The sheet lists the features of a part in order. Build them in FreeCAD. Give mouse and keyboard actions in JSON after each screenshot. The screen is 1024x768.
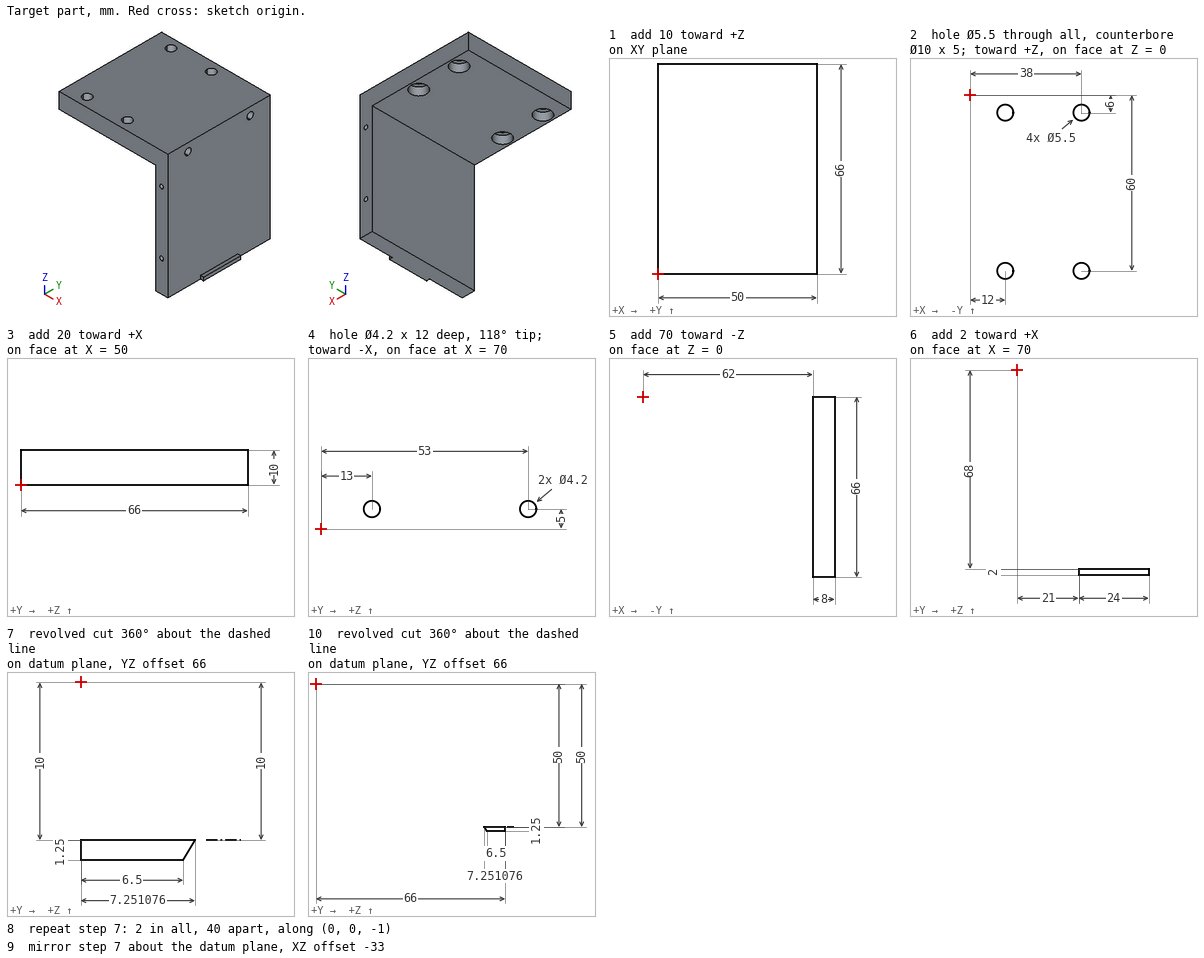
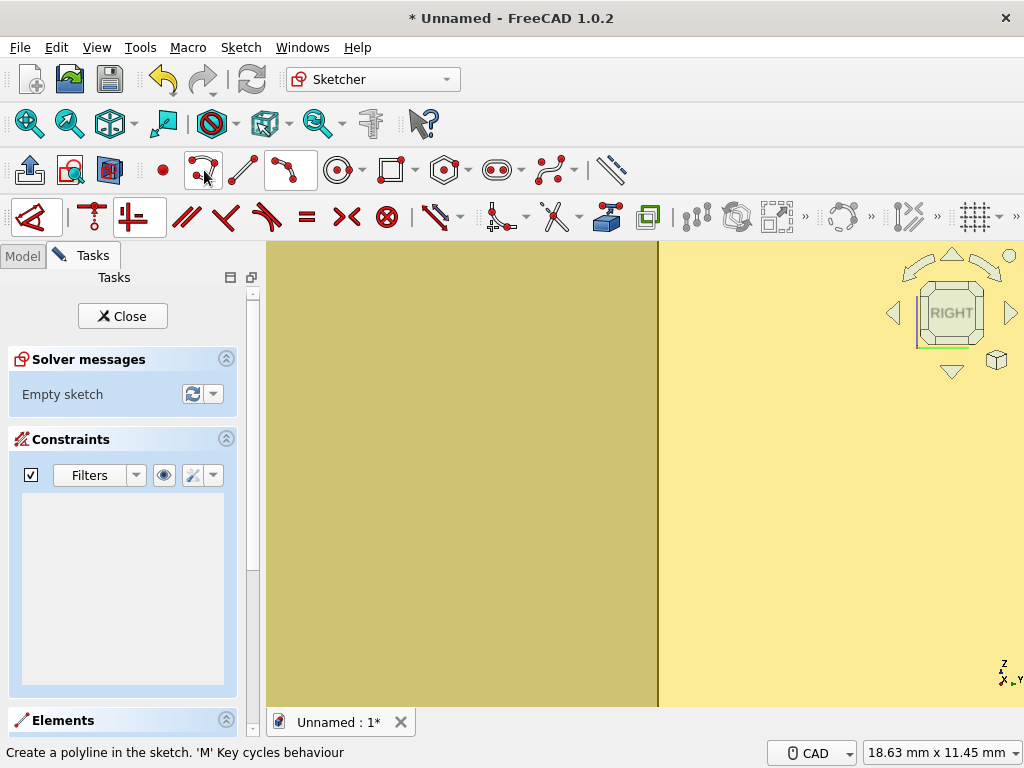
{"action": "left_click", "coordinate": [363, 439]}
{"action": "left_click", "coordinate": [393, 490]}
{"action": "left_click", "coordinate": [658, 490]}
{"action": "left_click", "coordinate": [658, 439]}
{"action": "left_click", "coordinate": [363, 440]}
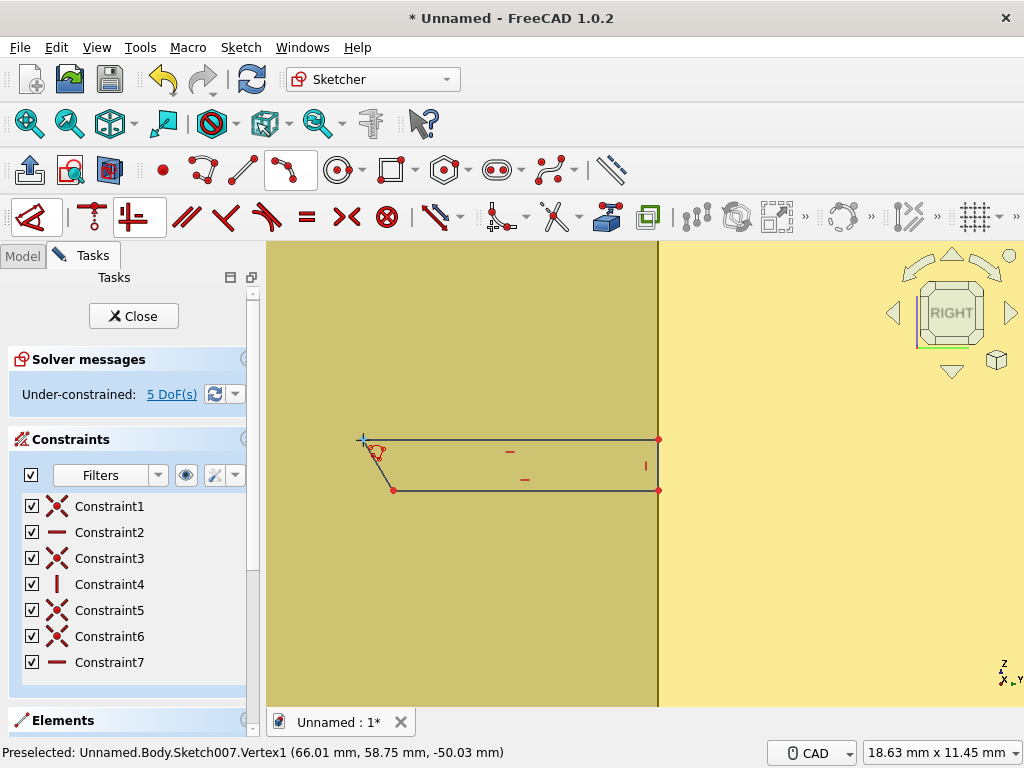
{"action": "key", "text": "g l"}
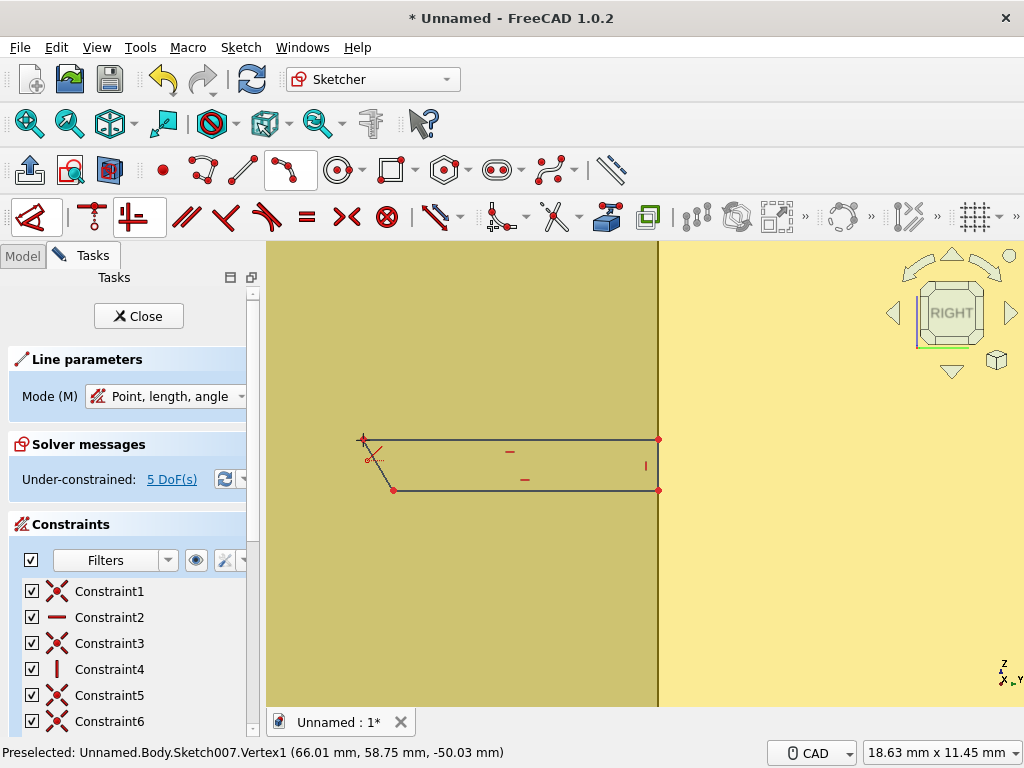
{"action": "left_click", "coordinate": [687, 439]}
{"action": "left_click", "coordinate": [776, 439]}
{"action": "key", "text": "Escape"}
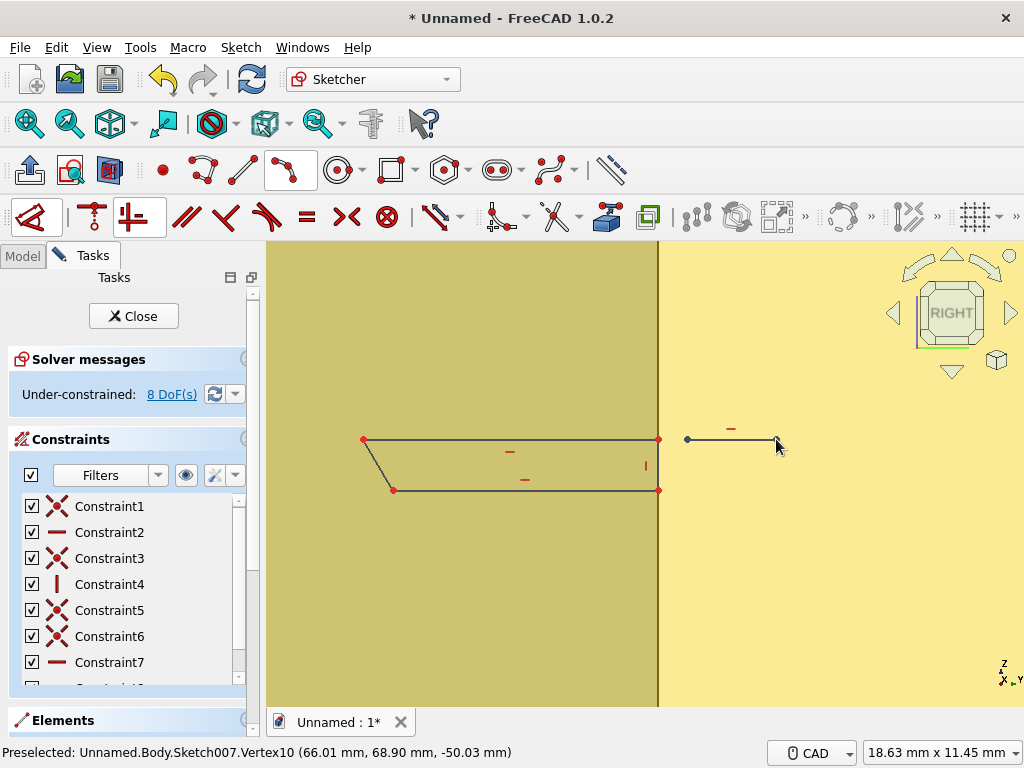
{"action": "left_click", "coordinate": [714, 440]}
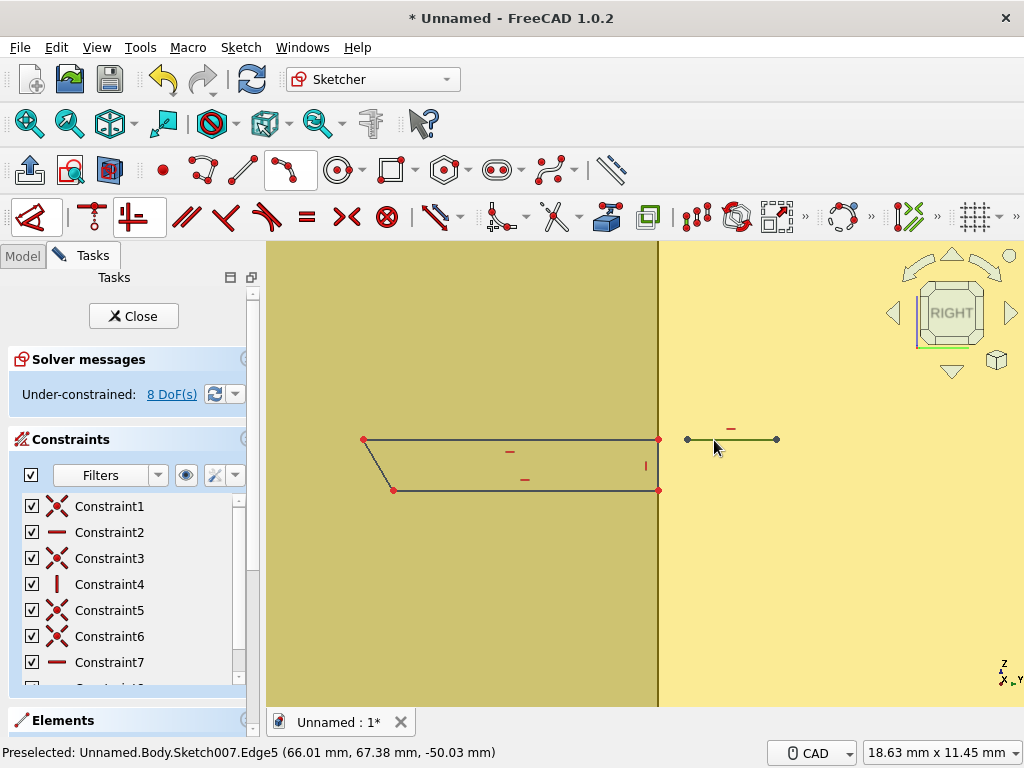
{"action": "key", "text": "g n"}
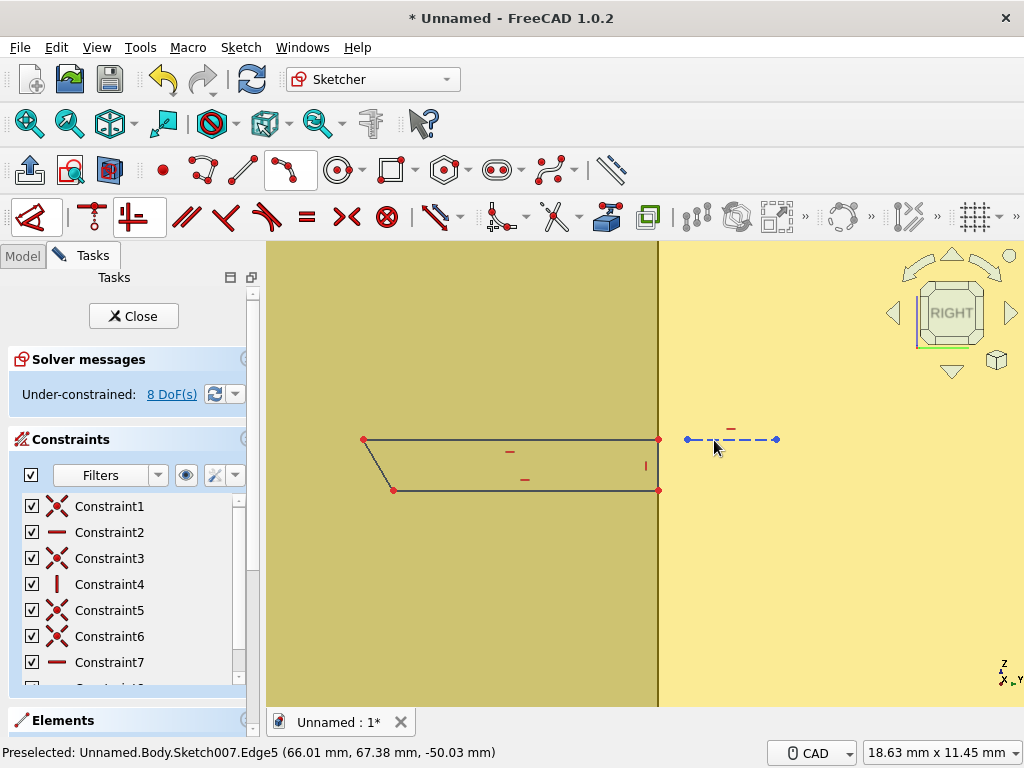
{"action": "left_click", "coordinate": [472, 491]}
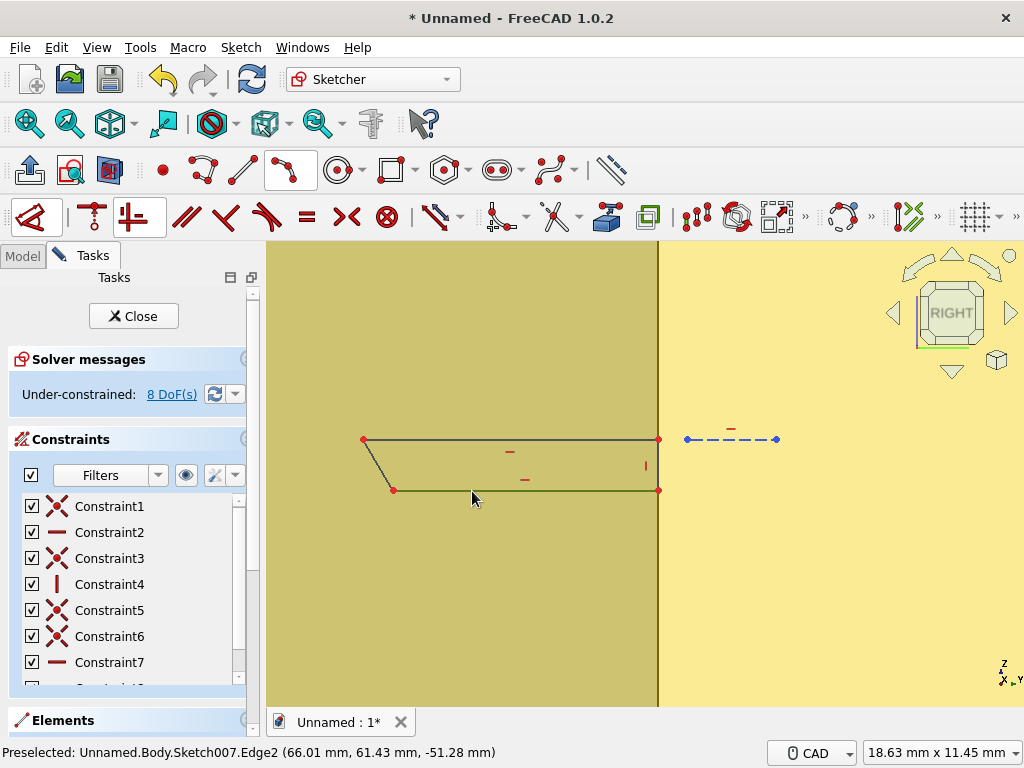
{"action": "key", "text": "l"}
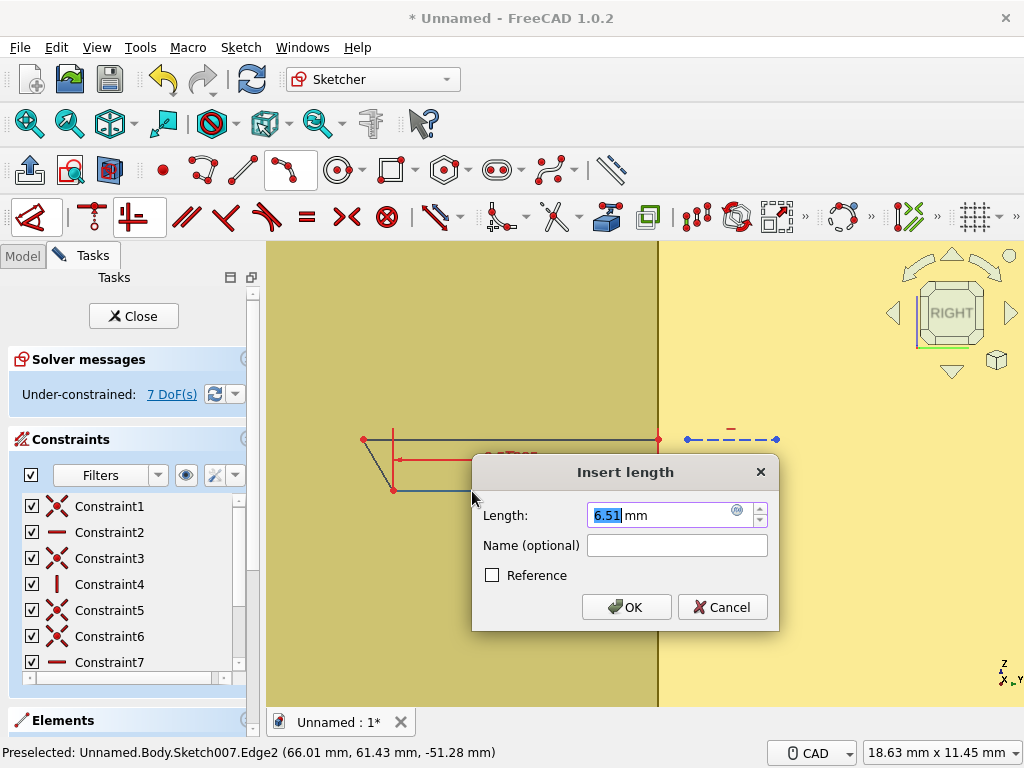
{"action": "type", "text": "6.5"}
{"action": "key", "text": "Return"}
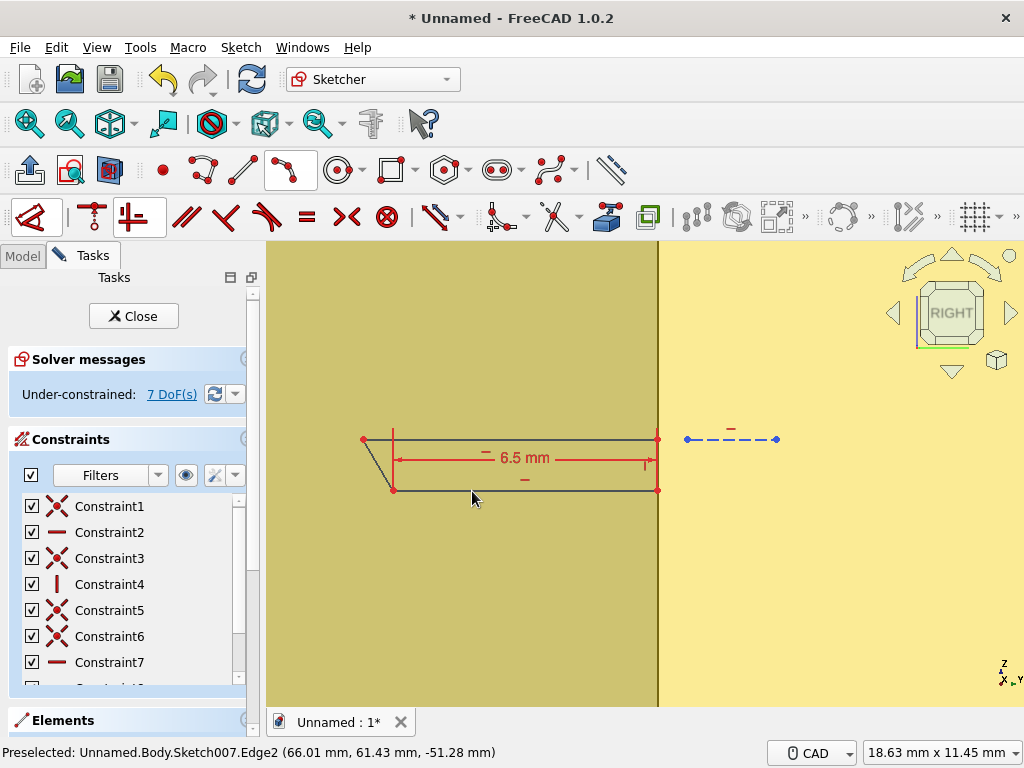
{"action": "left_click", "coordinate": [363, 440]}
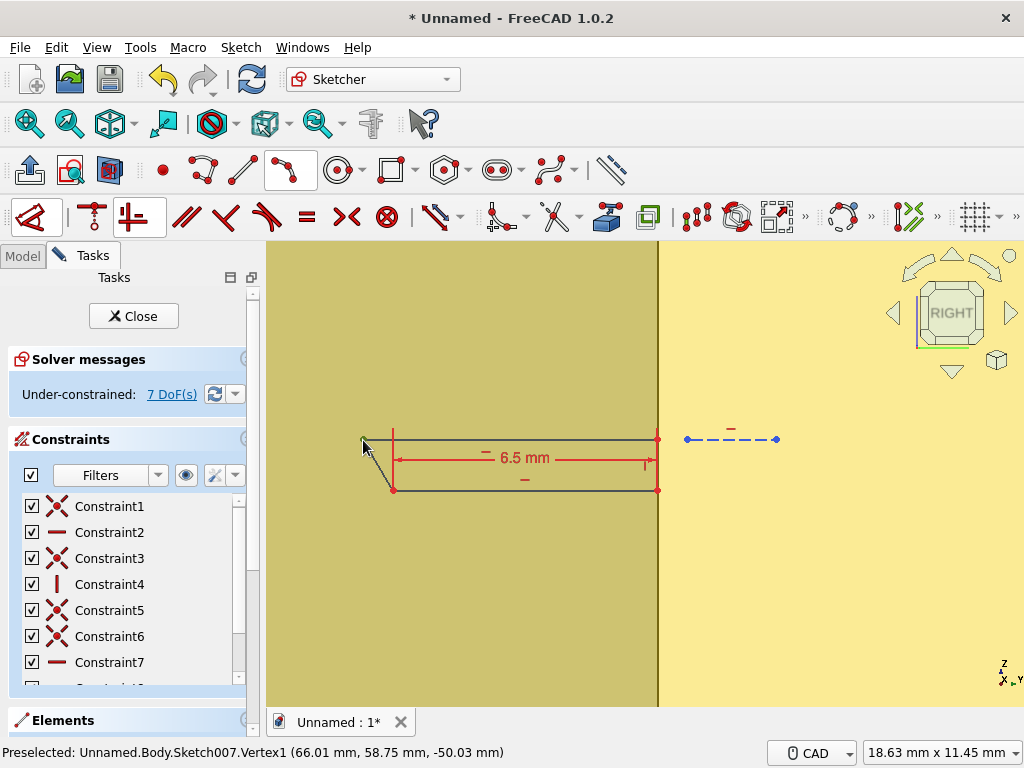
{"action": "key", "text": "i"}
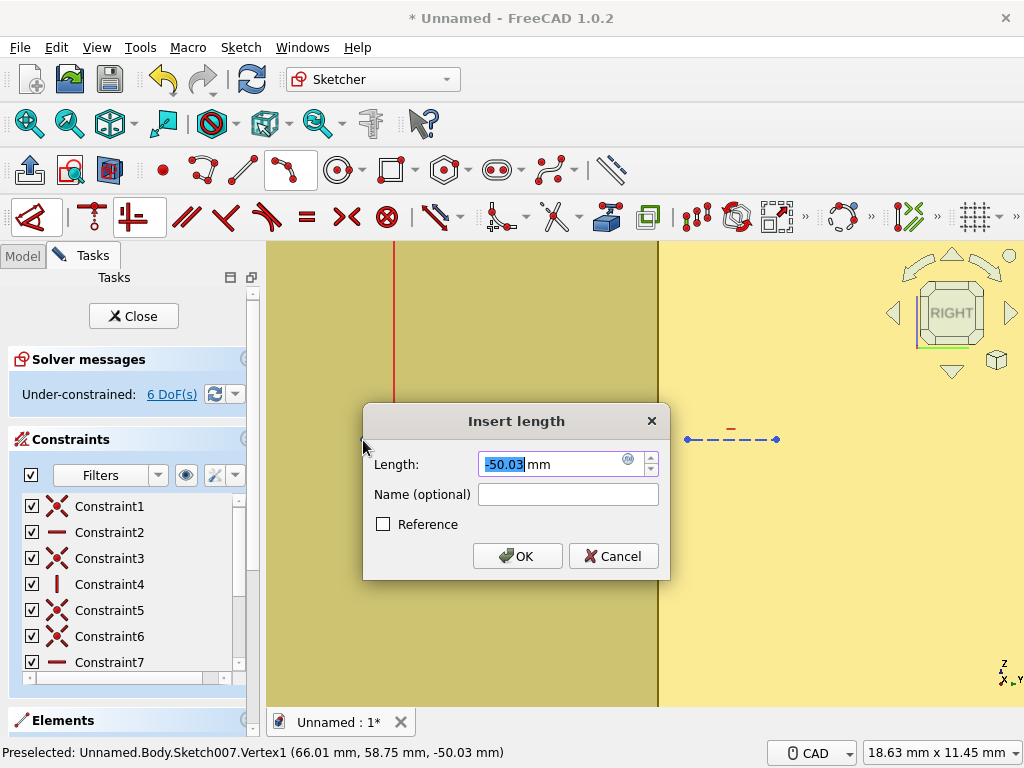
{"action": "type", "text": "-50"}
{"action": "key", "text": "Return"}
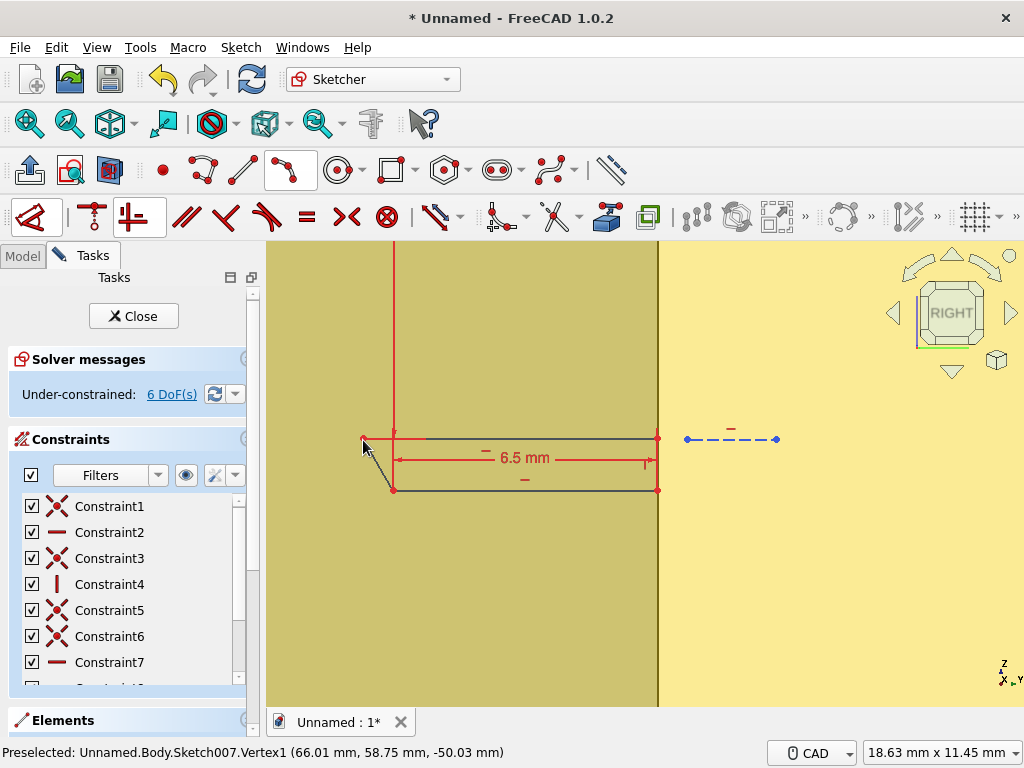
{"action": "left_click", "coordinate": [657, 491]}